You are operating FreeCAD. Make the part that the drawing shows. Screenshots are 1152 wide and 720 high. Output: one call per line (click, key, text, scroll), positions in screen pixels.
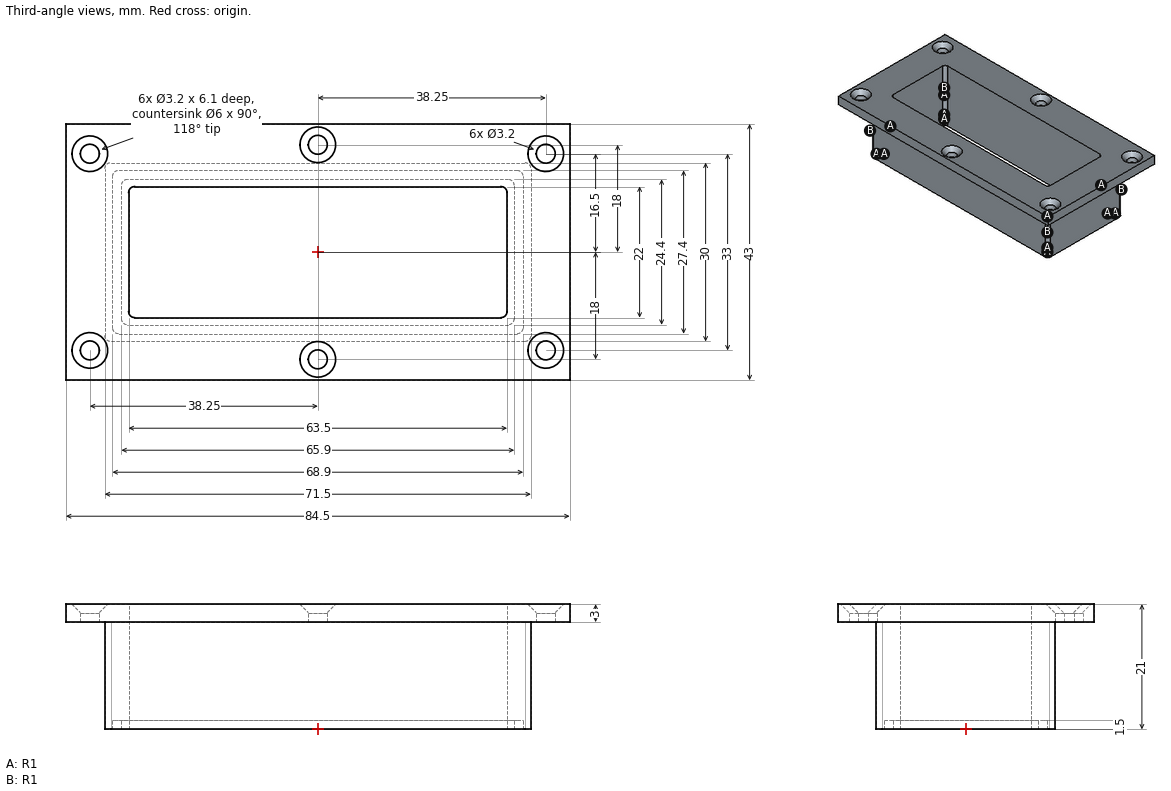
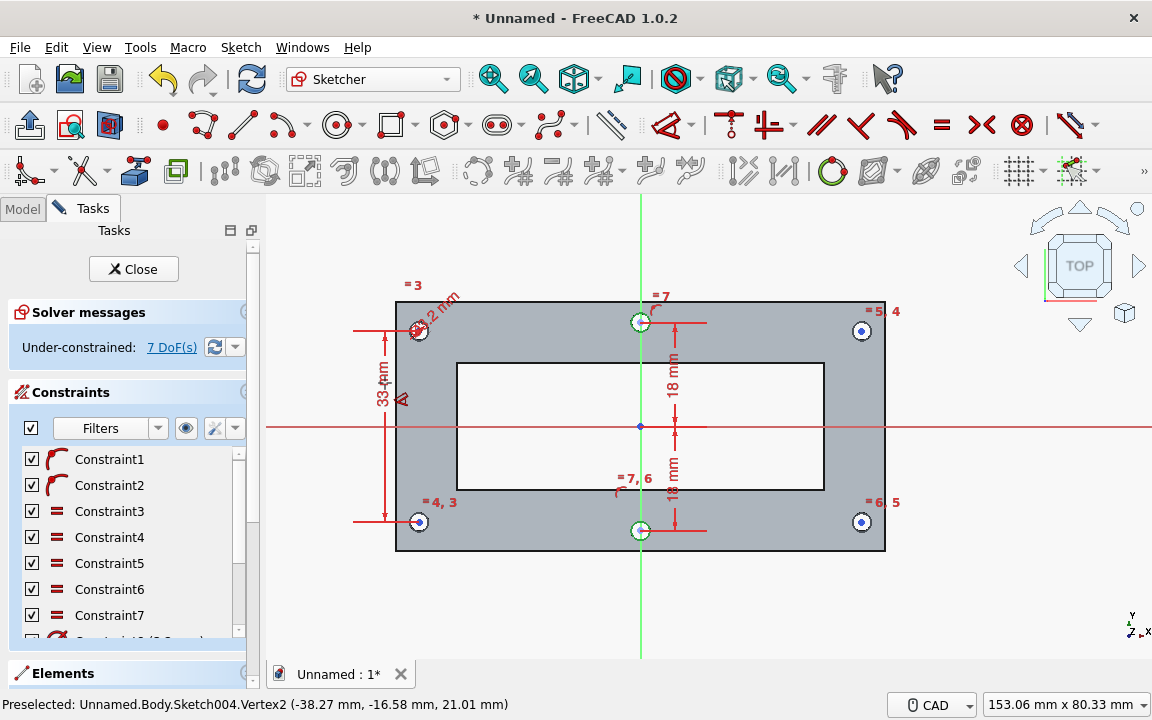
click(419, 522)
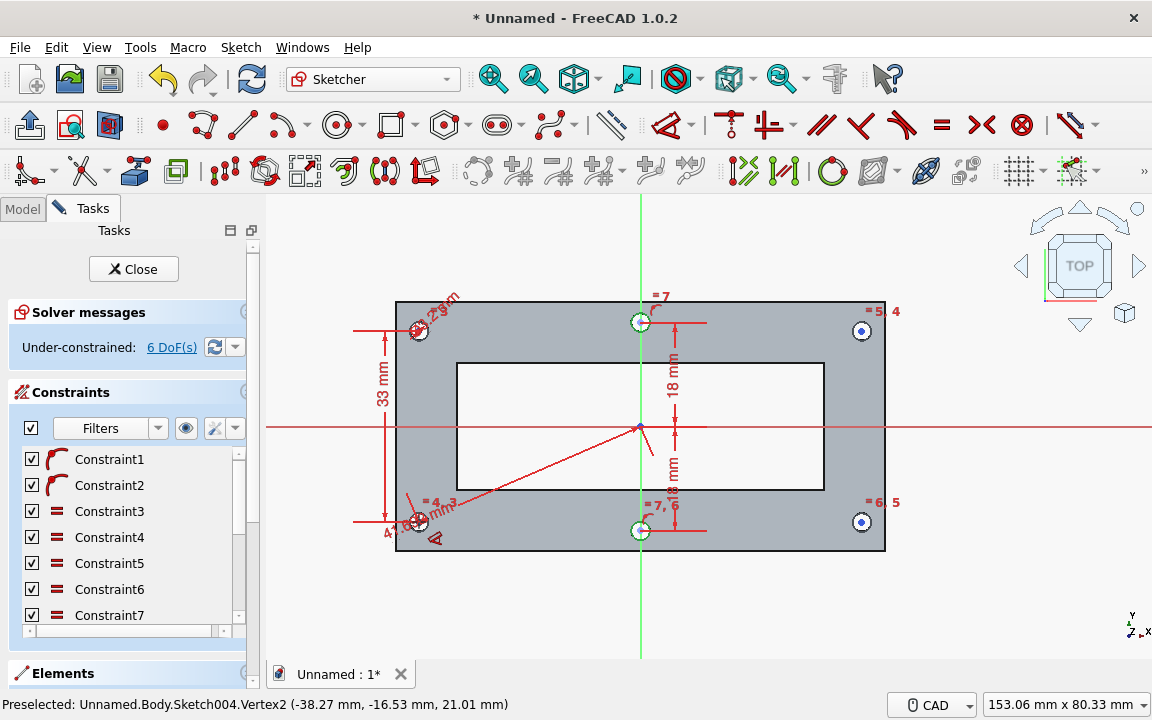
click(862, 331)
click(385, 471)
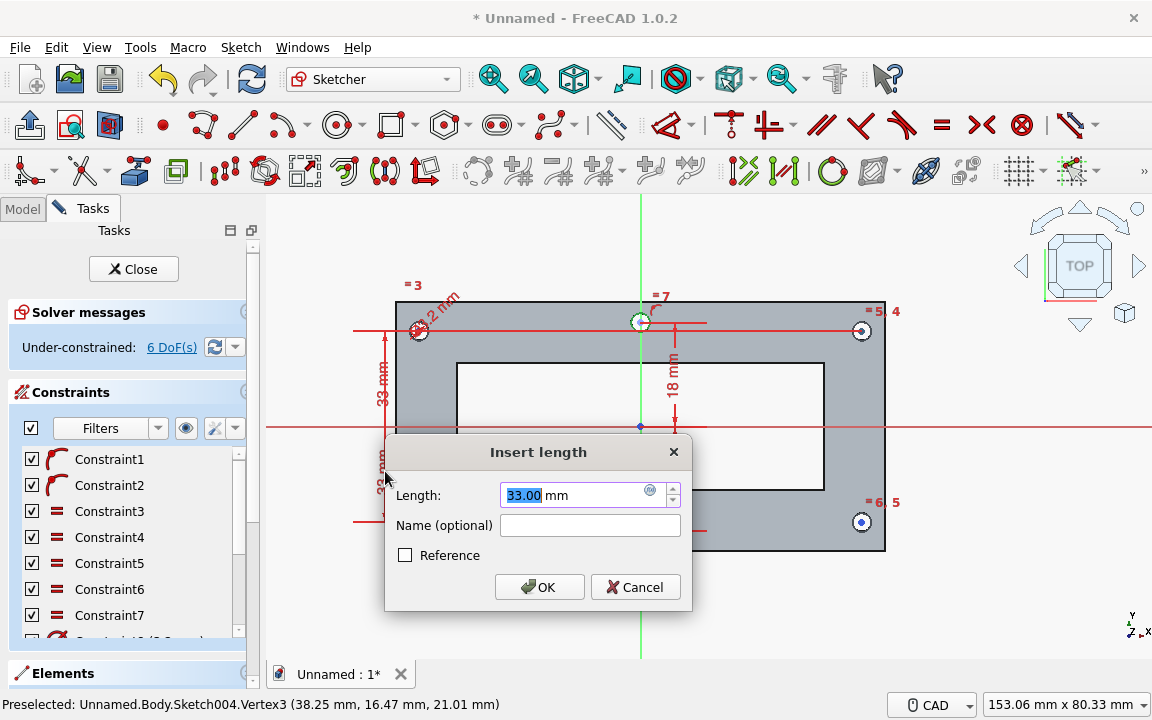
text(33)
key(Return)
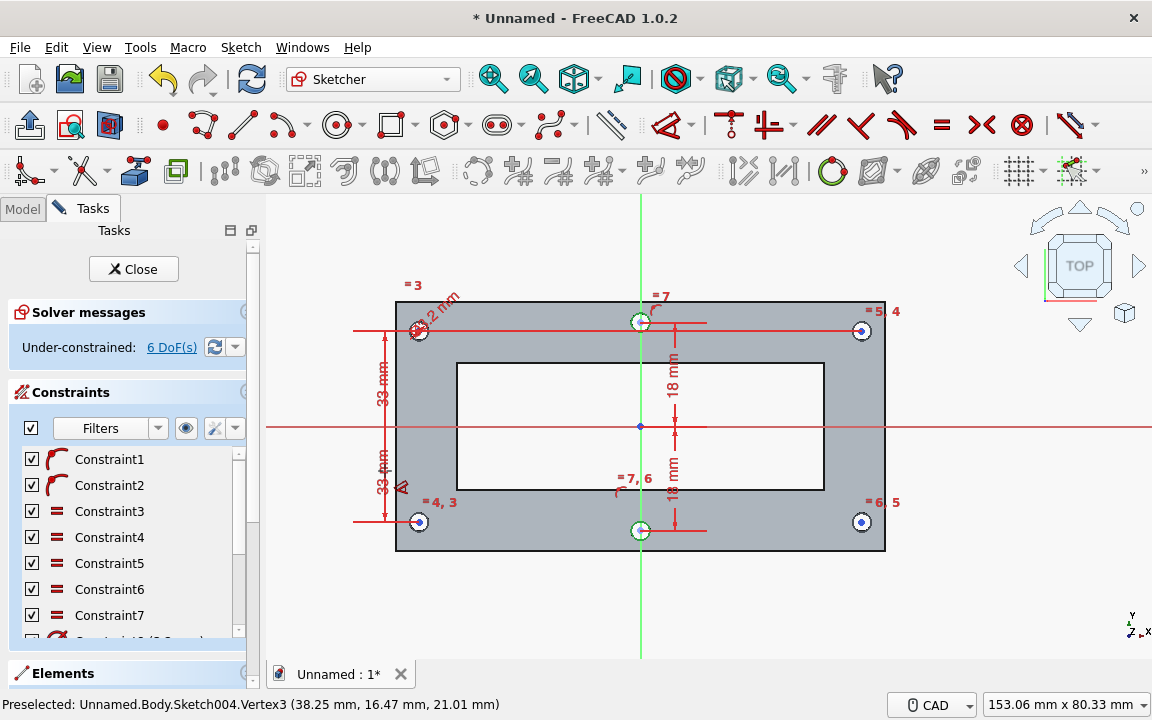
click(862, 331)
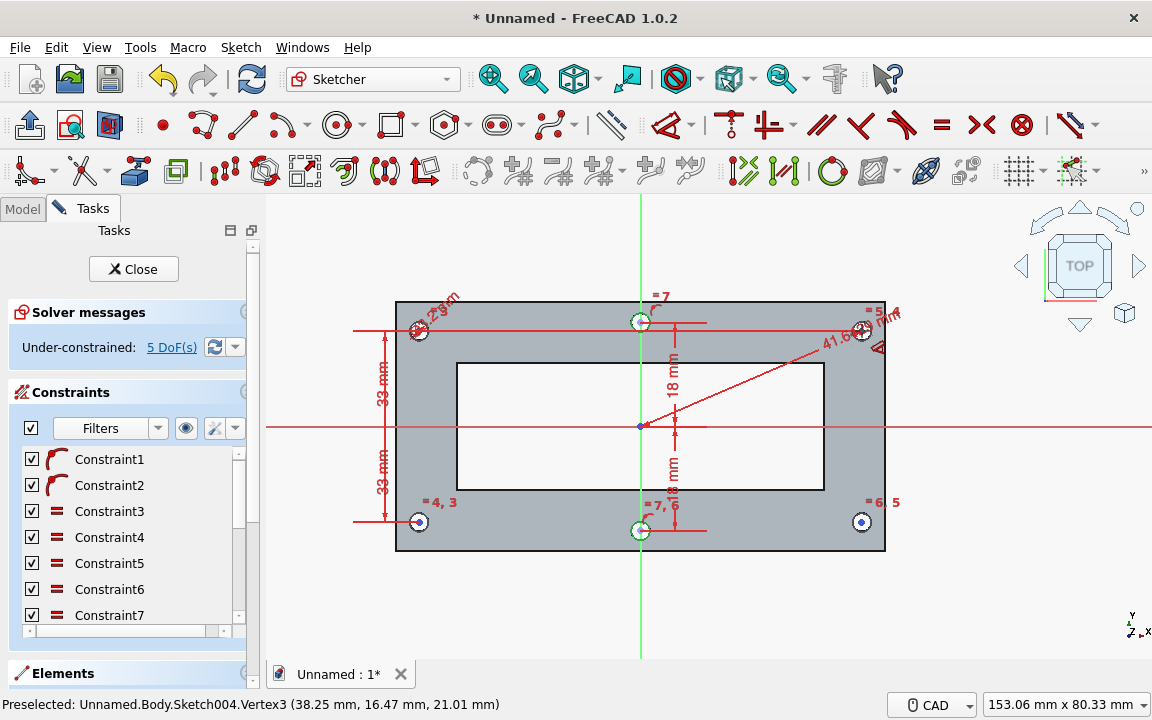
click(862, 523)
click(896, 383)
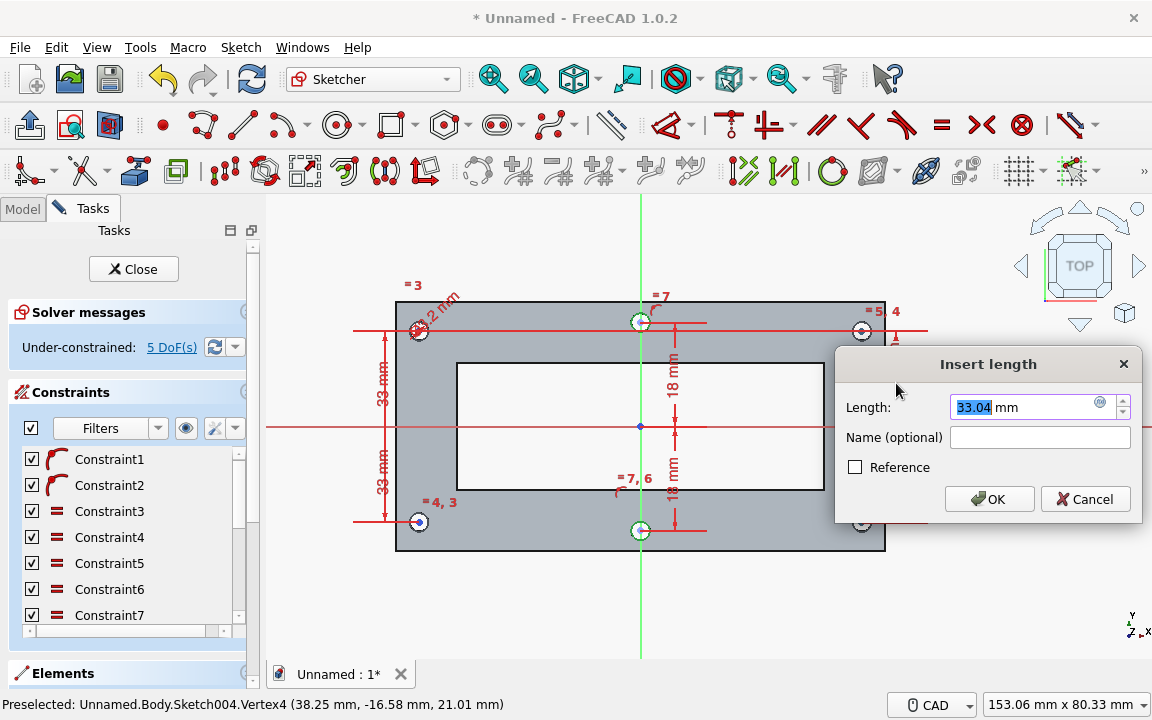
text(33)
key(Return)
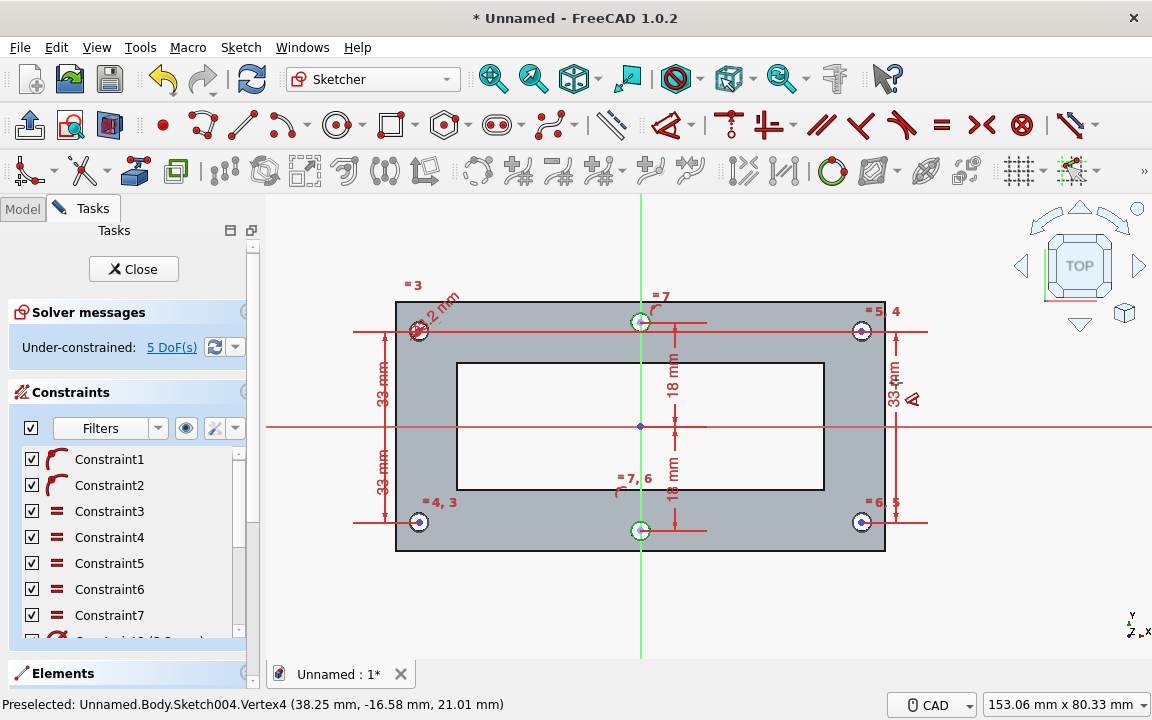
click(419, 332)
click(385, 357)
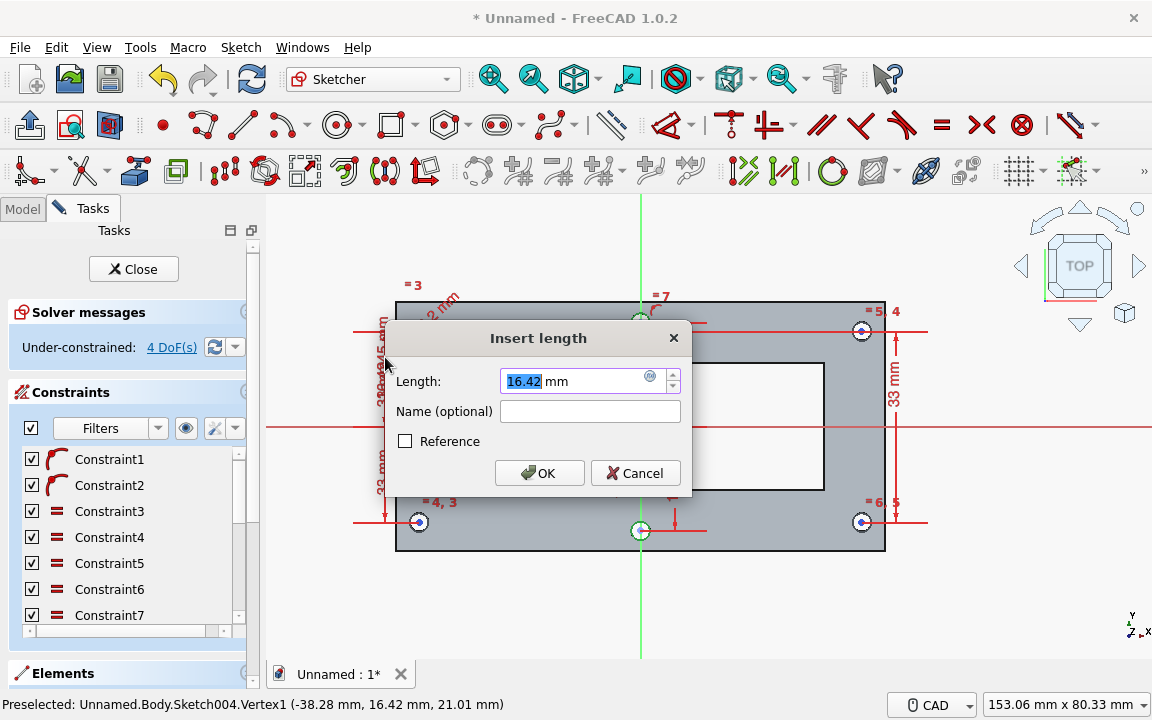
text(16.5)
key(Return)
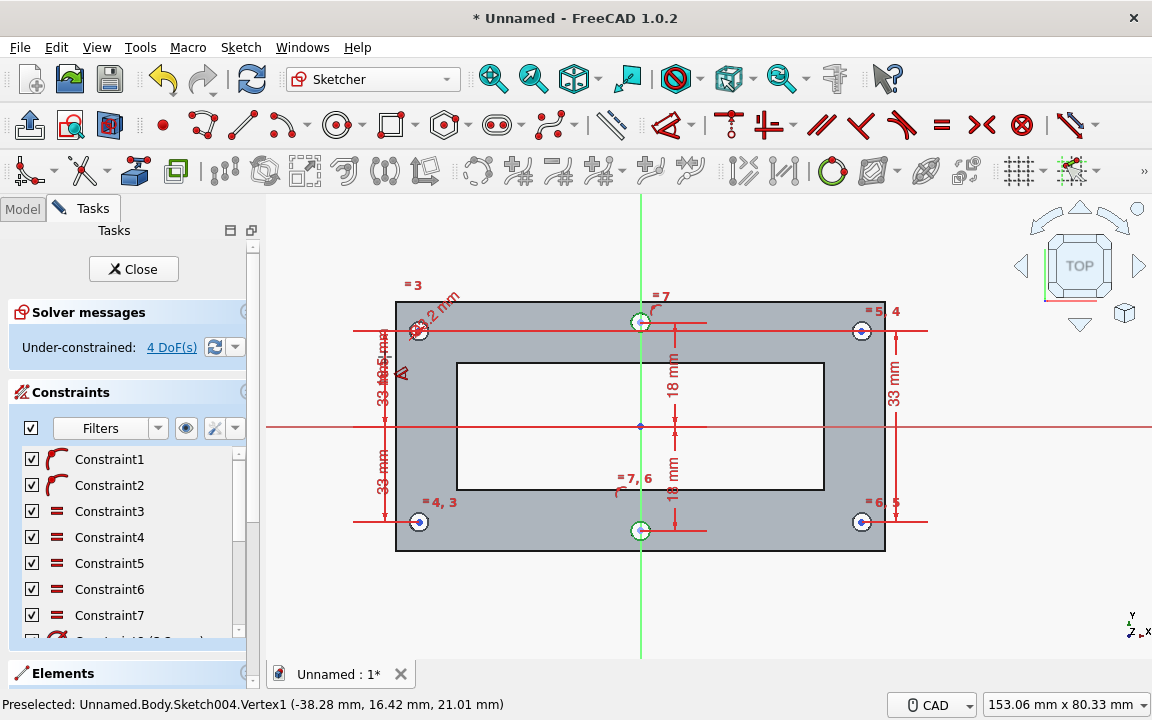
click(419, 331)
click(530, 297)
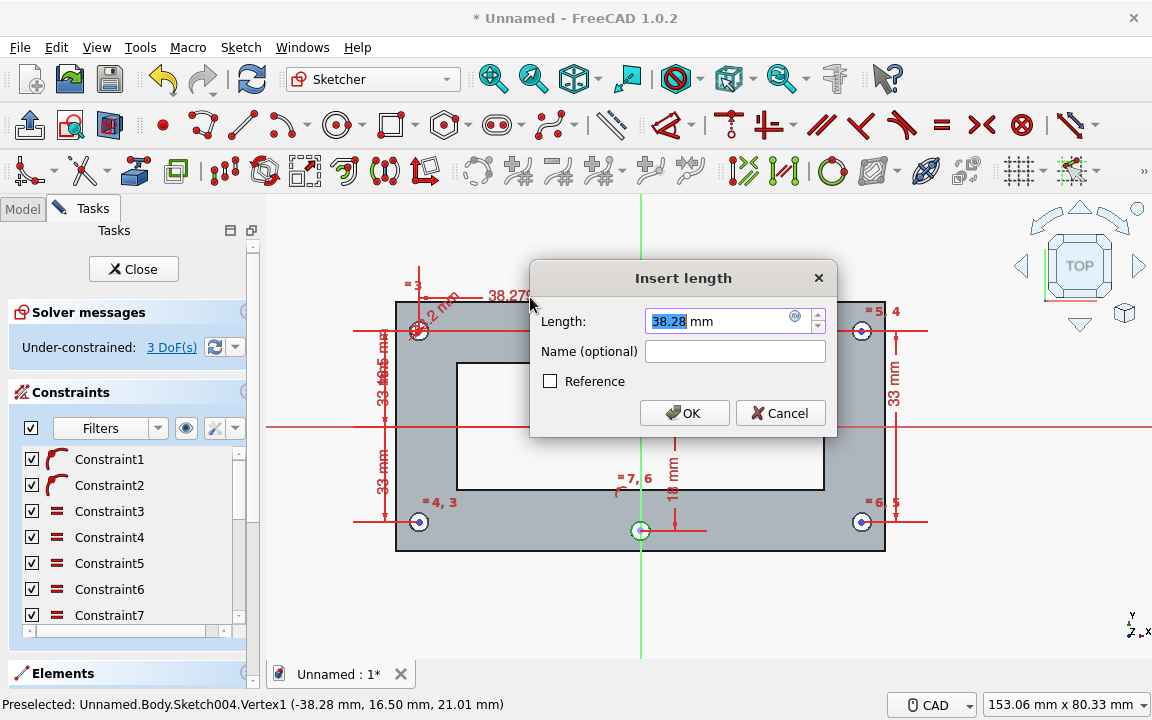
text(38.25)
key(Return)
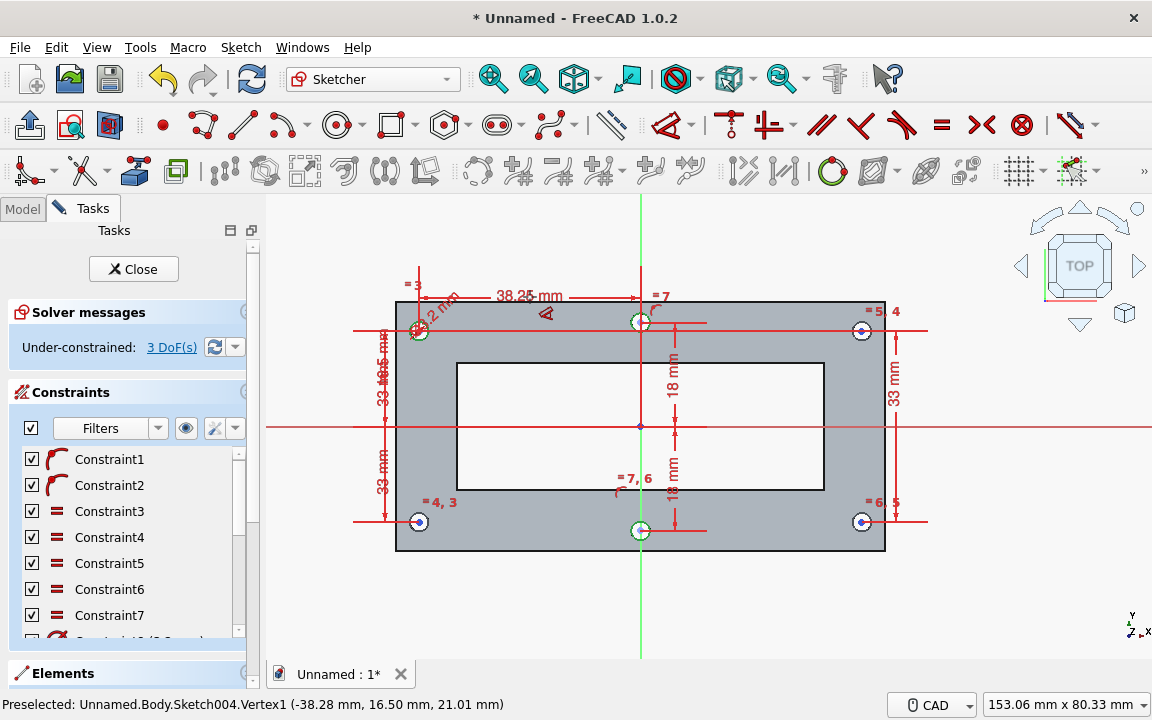
click(419, 522)
click(530, 556)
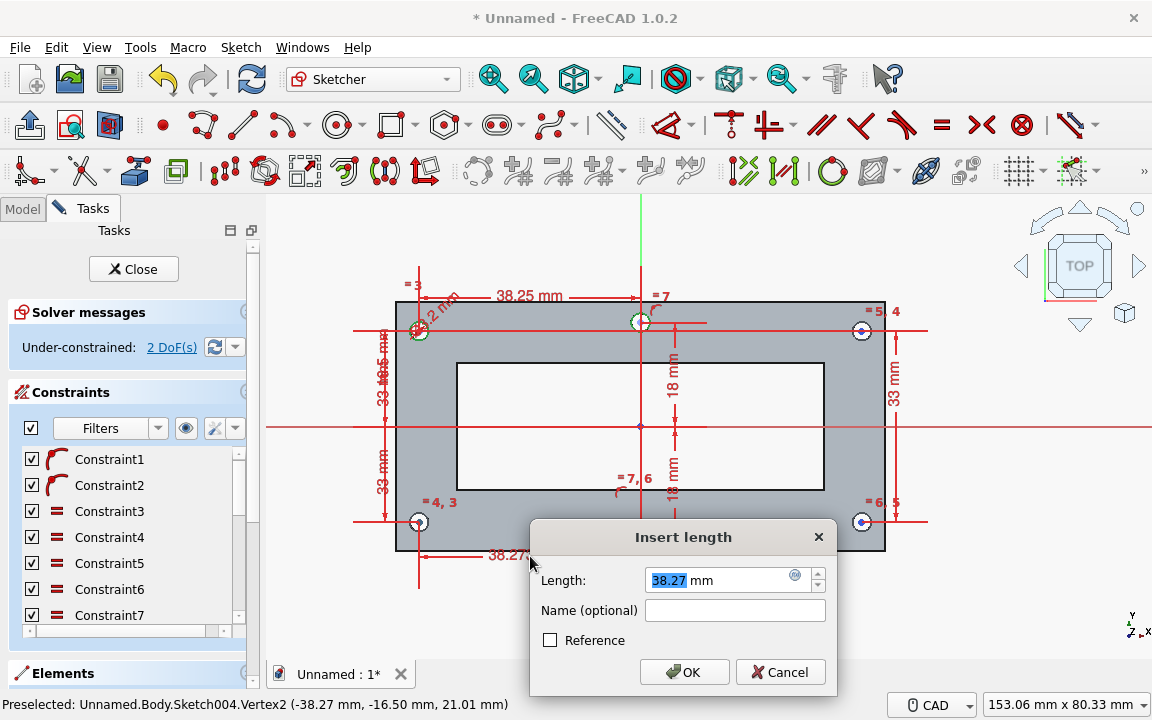
text(38.25)
key(Return)